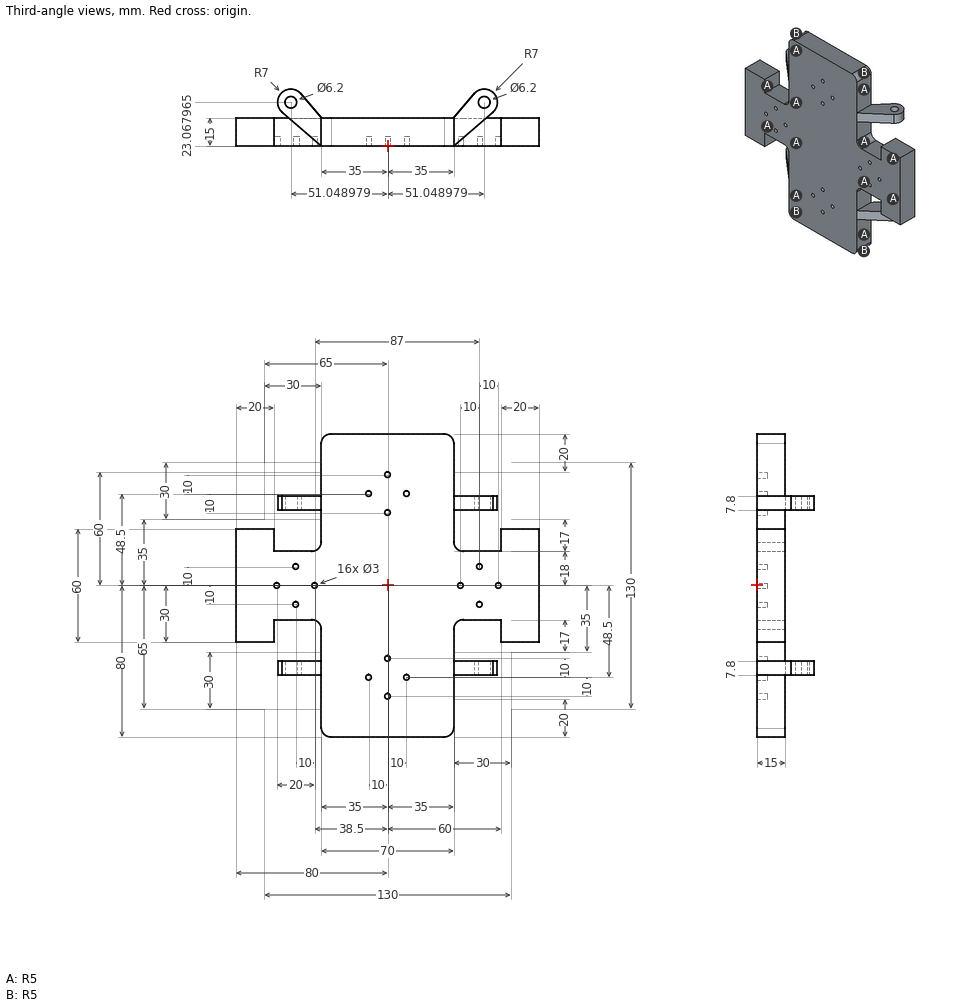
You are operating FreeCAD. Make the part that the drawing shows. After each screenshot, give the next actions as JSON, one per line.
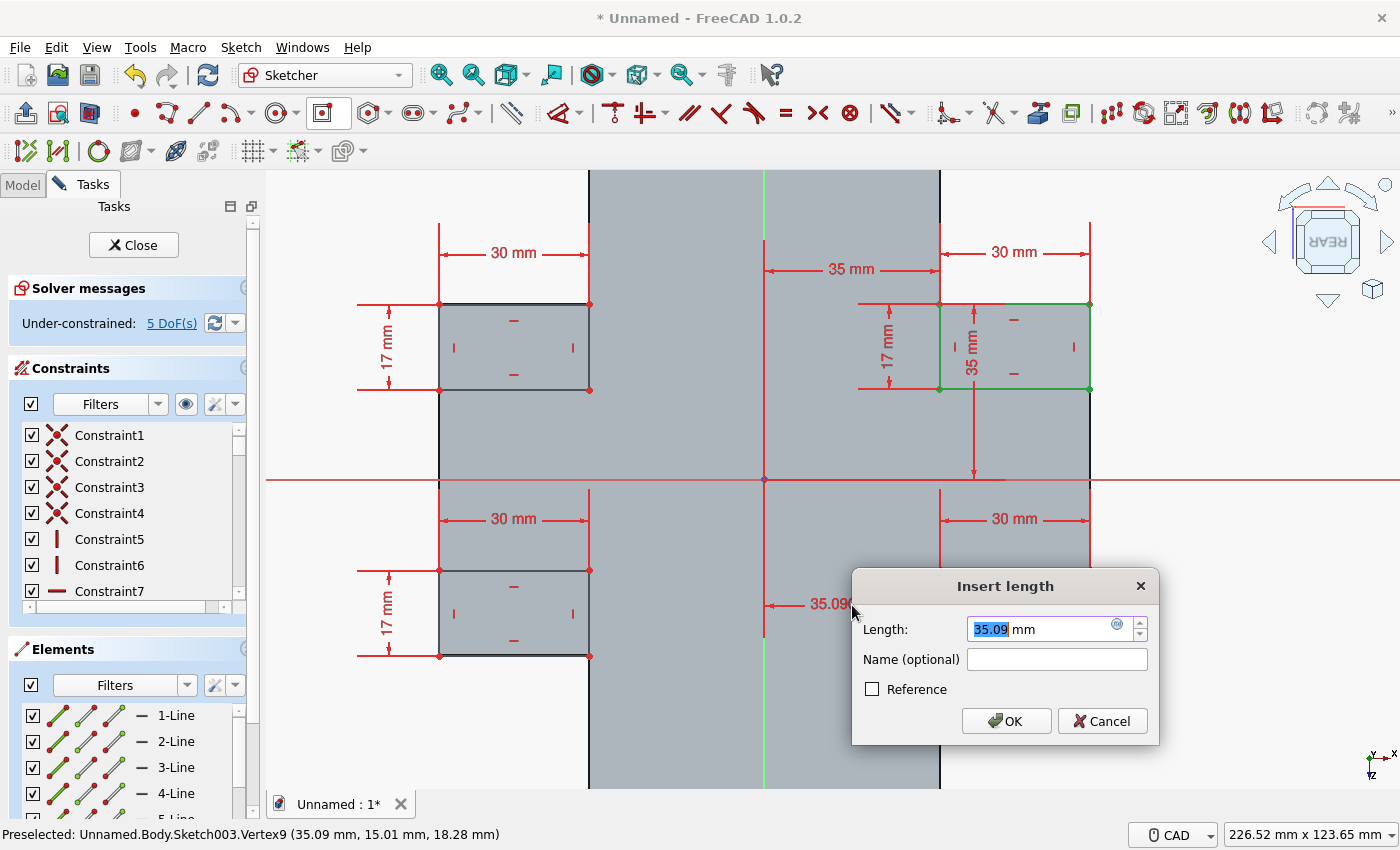
{"action": "type", "text": "35"}
{"action": "key", "text": "Return"}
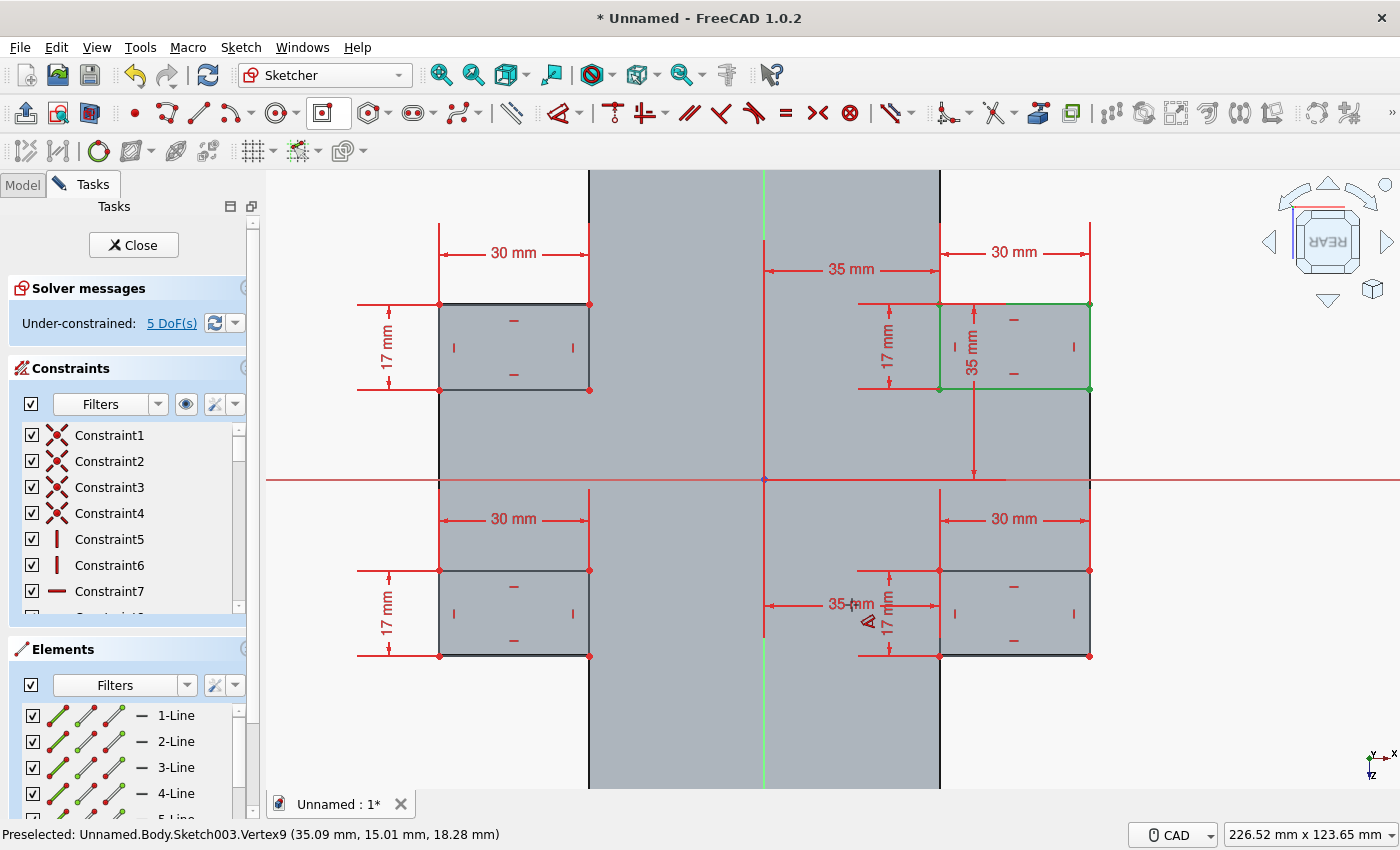
{"action": "left_click", "coordinate": [940, 571]}
{"action": "left_click", "coordinate": [974, 525]}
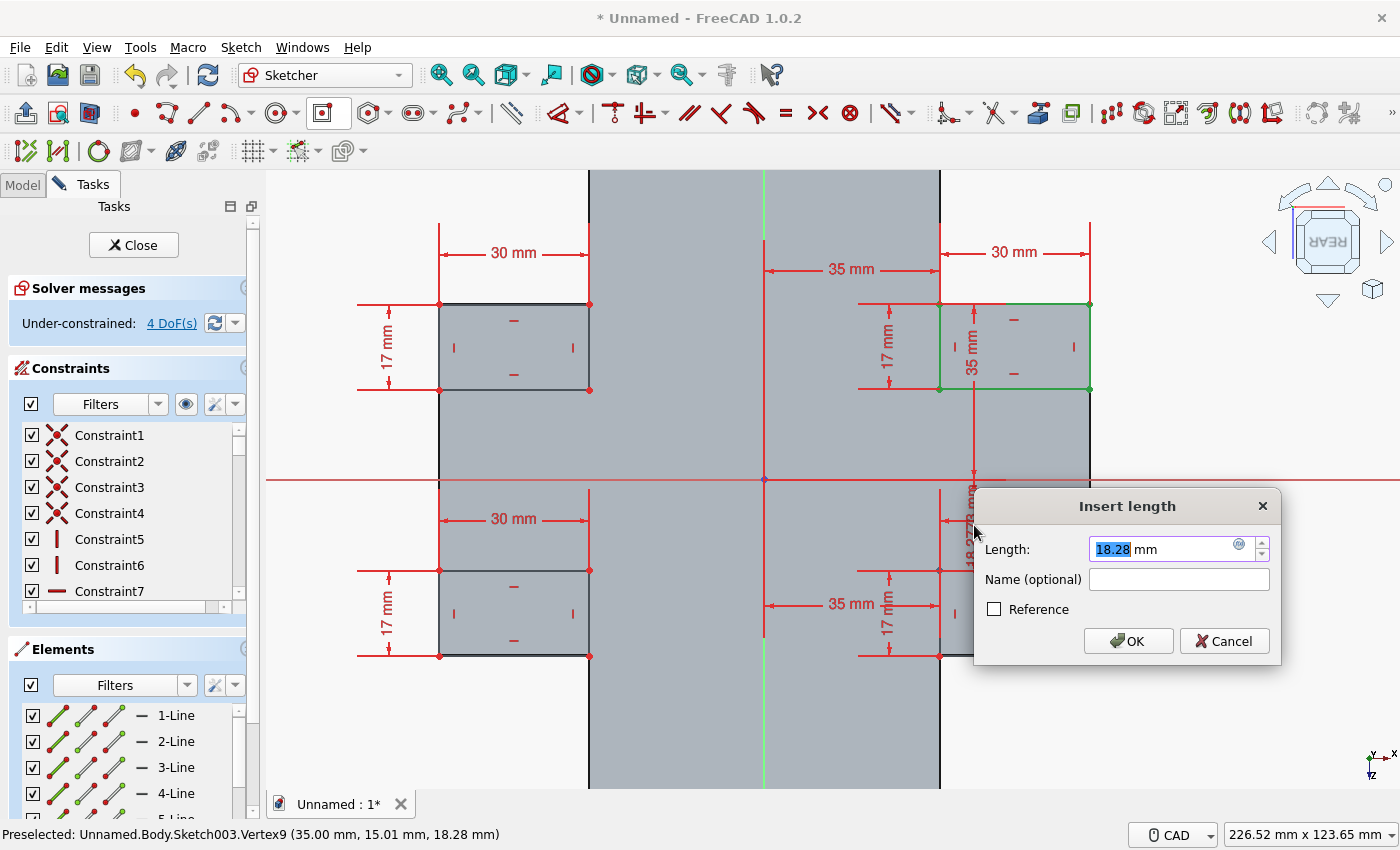
{"action": "type", "text": "18"}
{"action": "key", "text": "Return"}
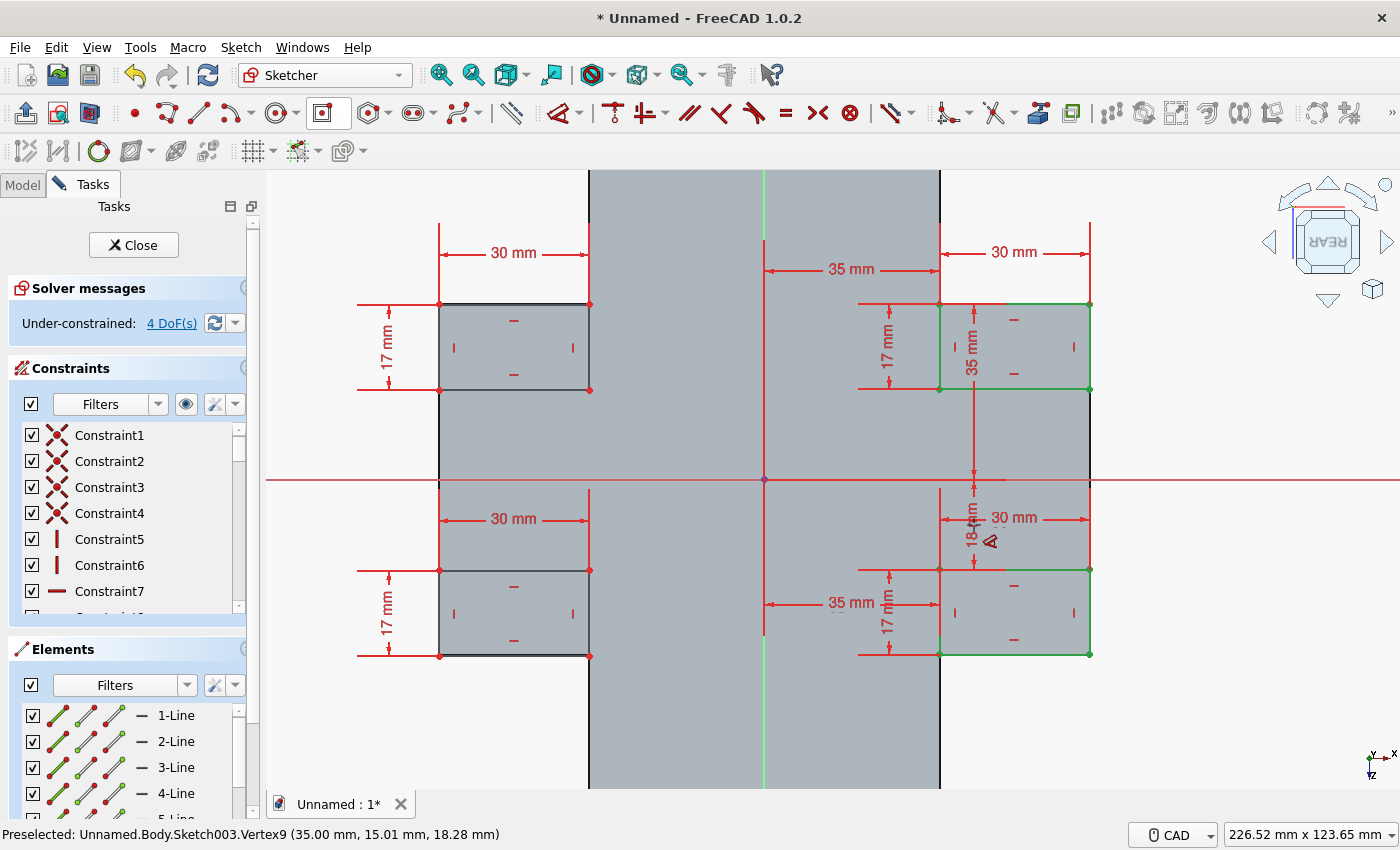
{"action": "left_click", "coordinate": [439, 305]}
{"action": "left_click", "coordinate": [602, 271]}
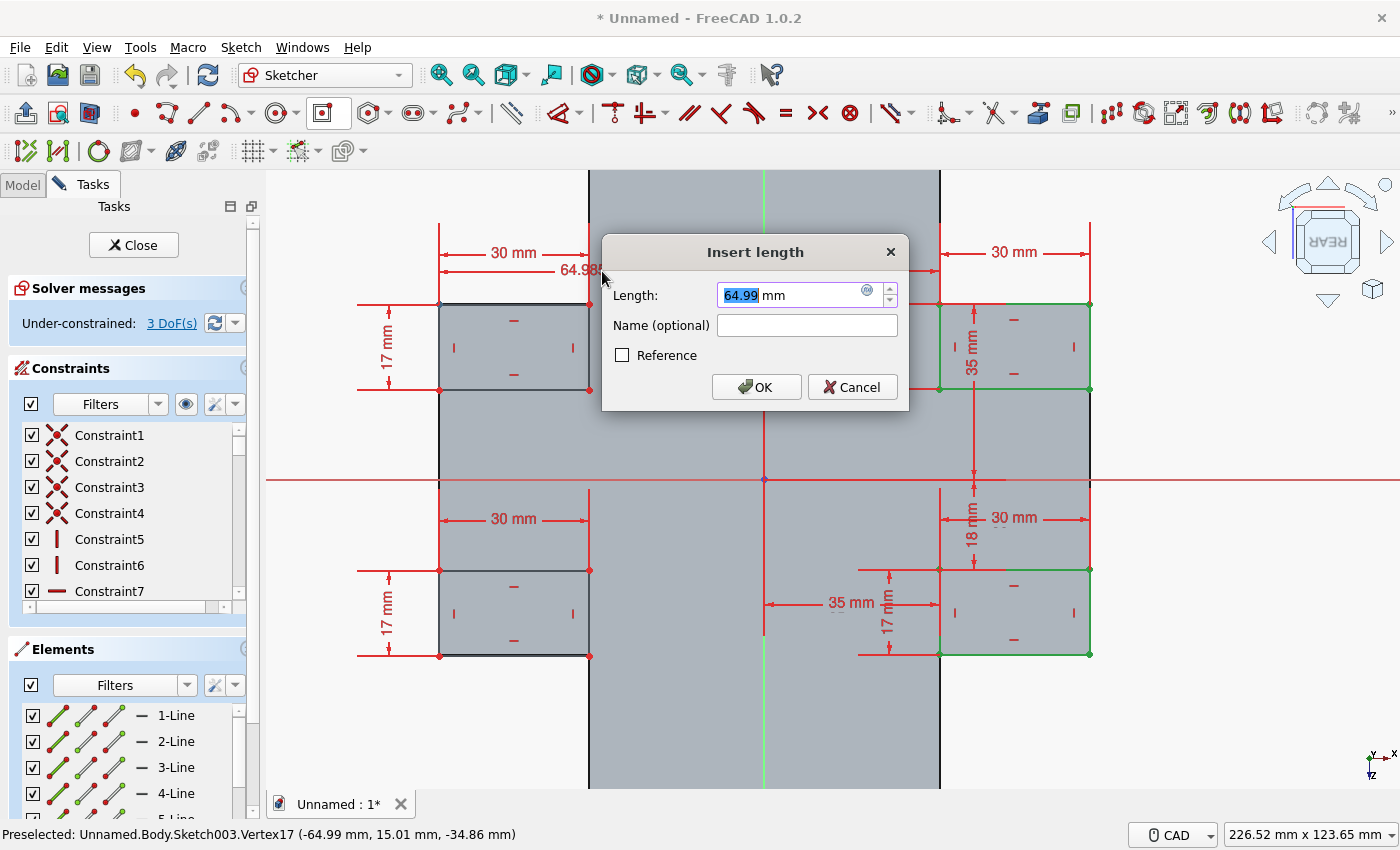
{"action": "type", "text": "65"}
{"action": "key", "text": "Return"}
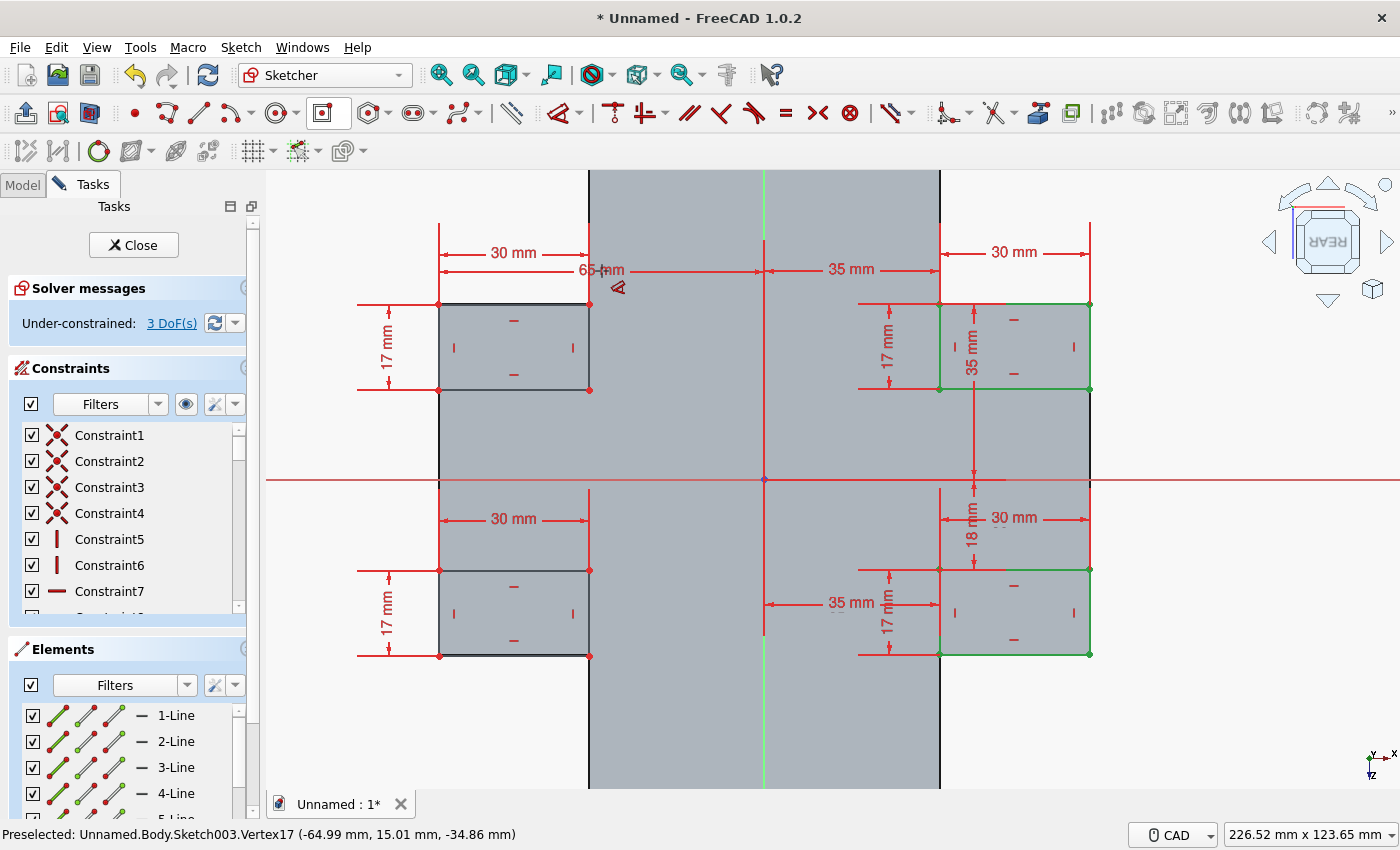
{"action": "left_click", "coordinate": [439, 305]}
{"action": "left_click", "coordinate": [405, 392]}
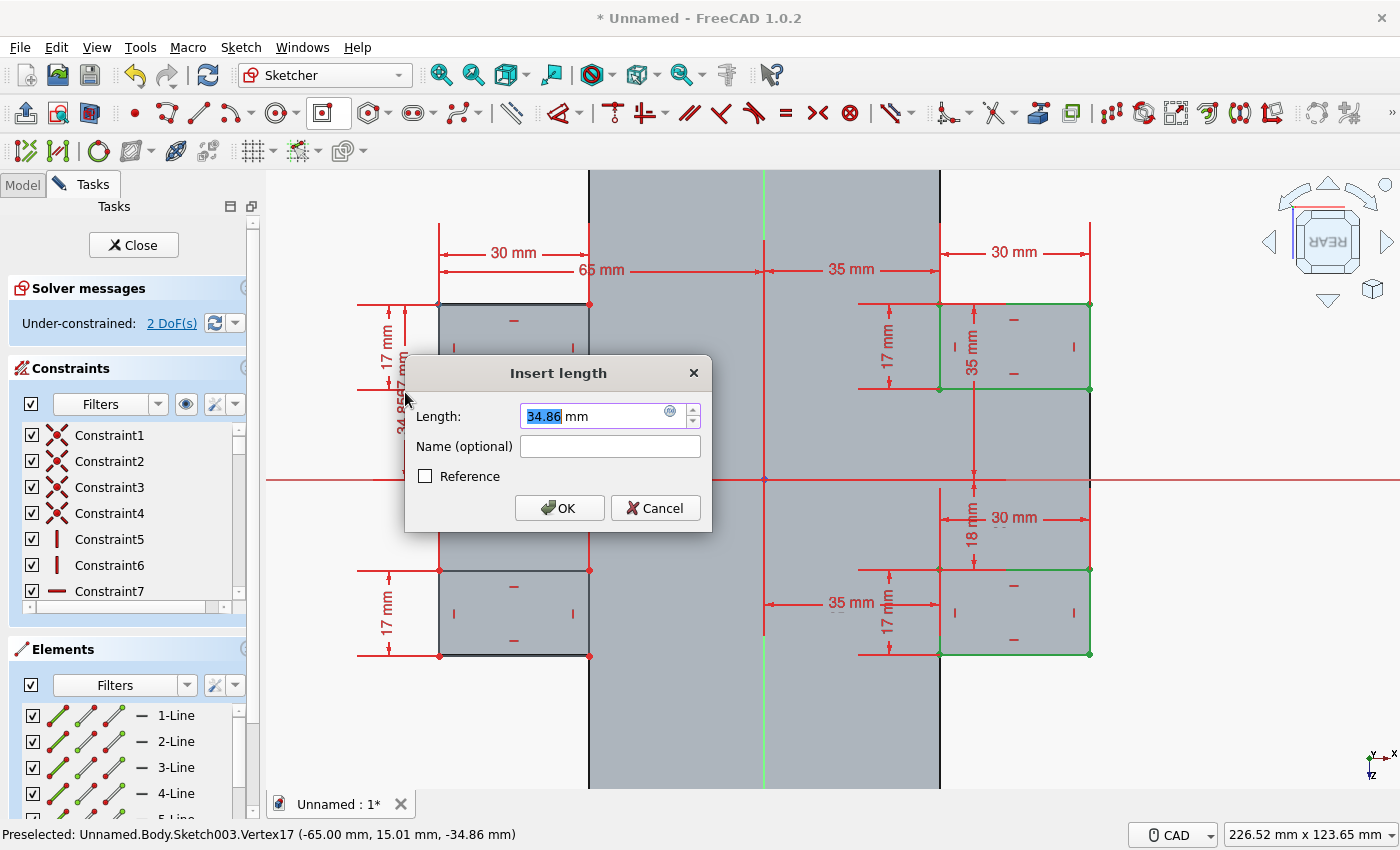
{"action": "type", "text": "35"}
{"action": "key", "text": "Return"}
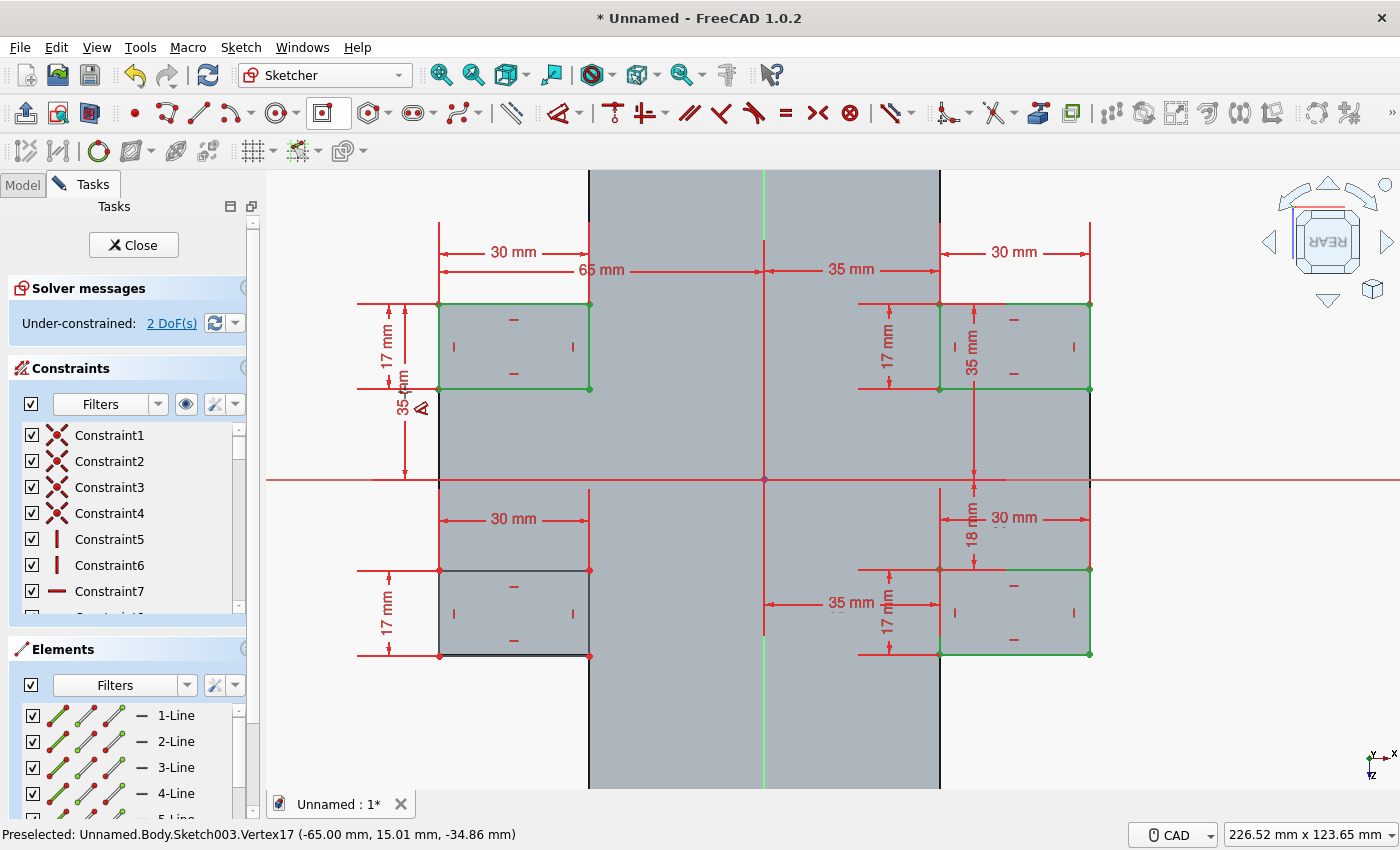
{"action": "left_click", "coordinate": [439, 571]}
{"action": "left_click", "coordinate": [527, 605]}